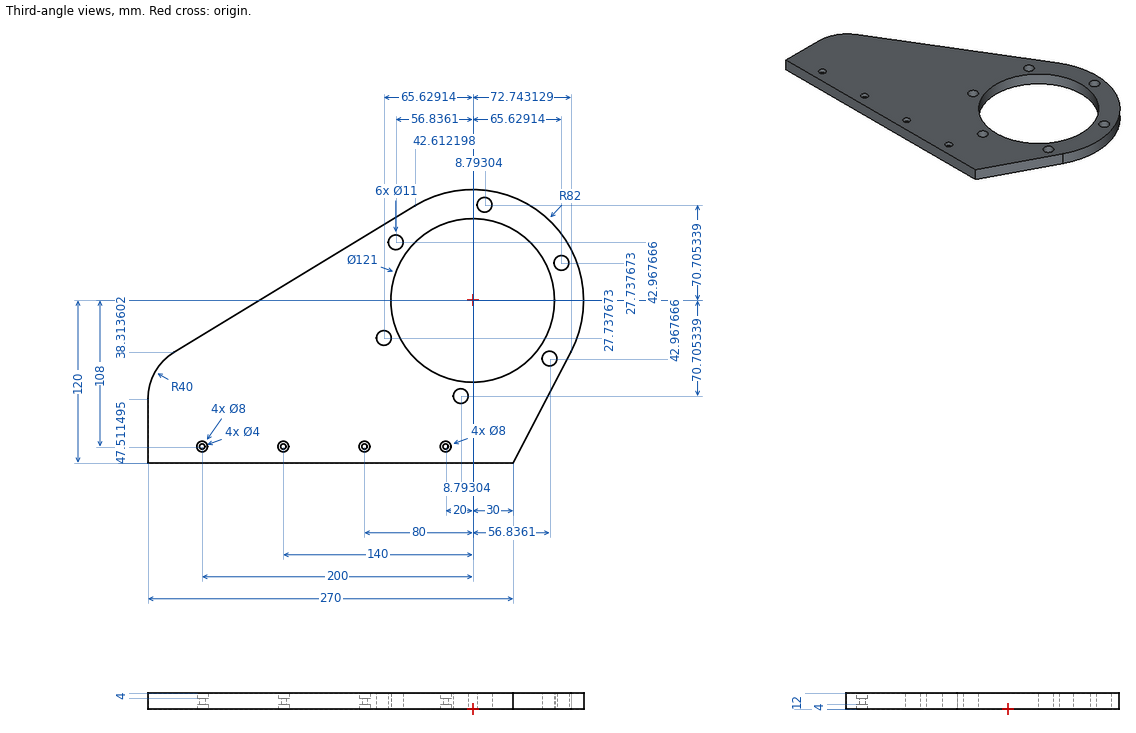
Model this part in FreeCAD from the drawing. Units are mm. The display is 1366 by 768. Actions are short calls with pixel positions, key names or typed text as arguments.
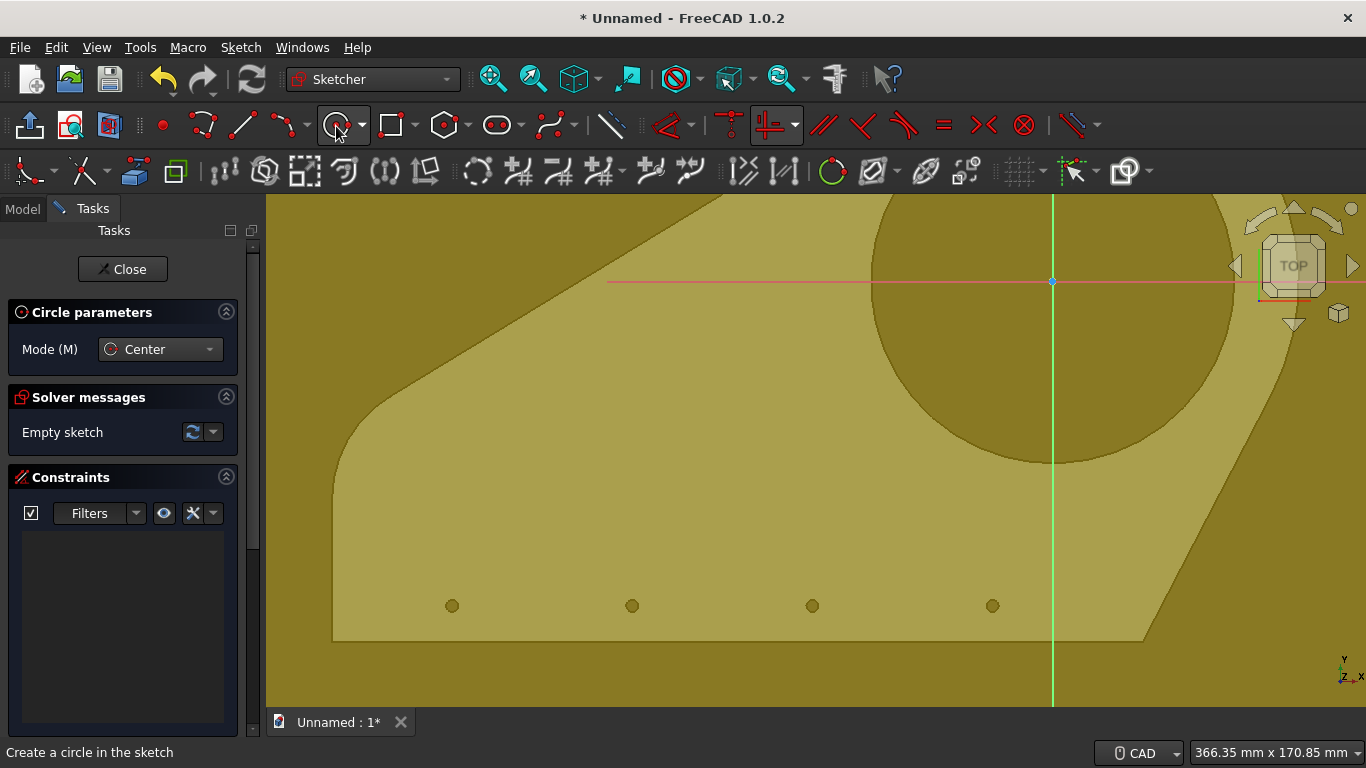
scroll(993, 606, up, 4)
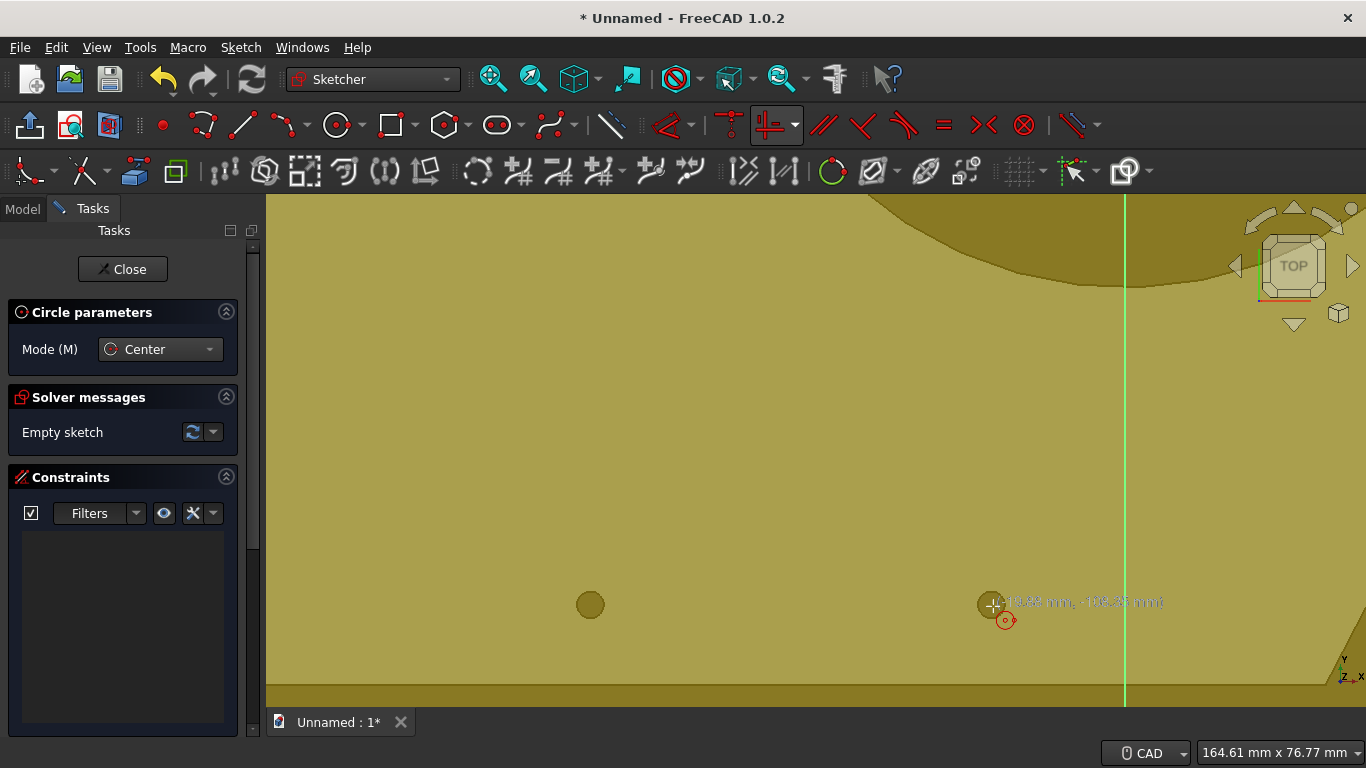
click(991, 605)
click(1010, 586)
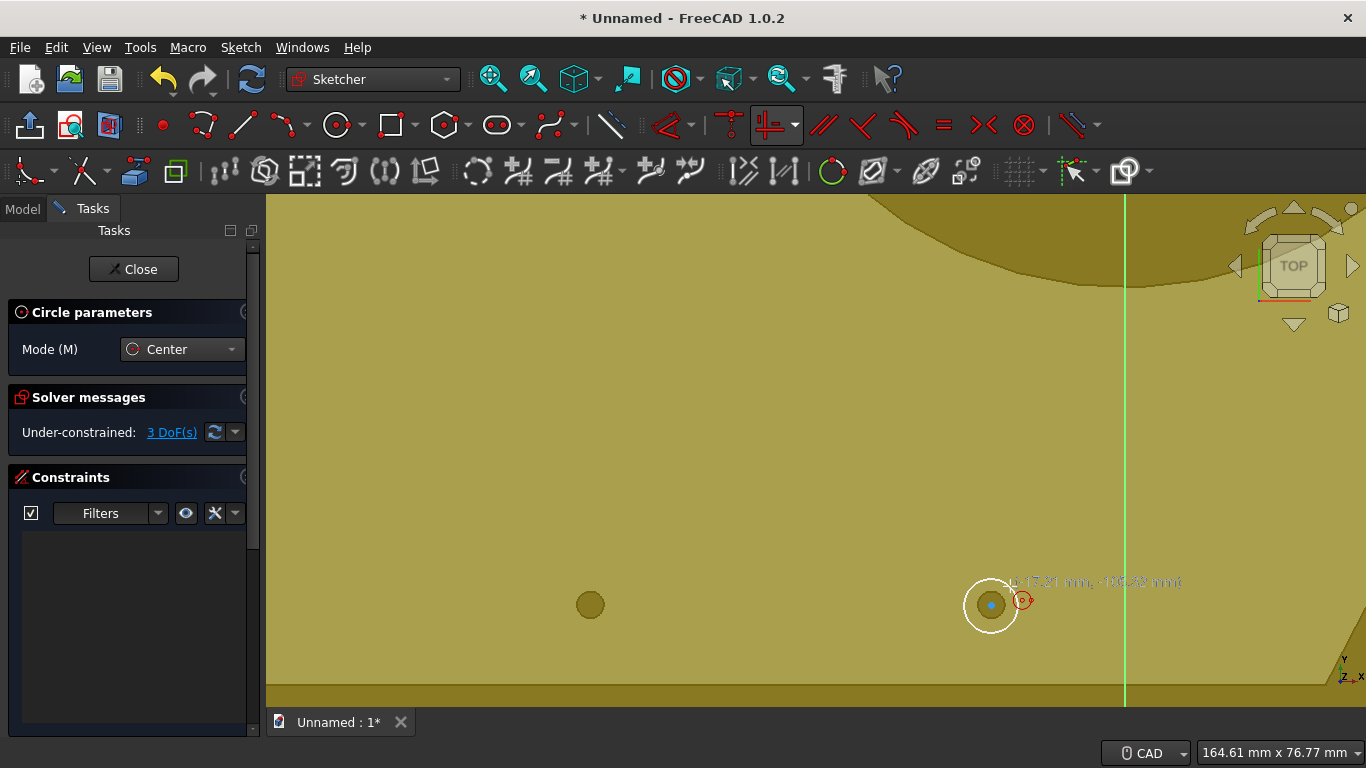
click(590, 605)
click(609, 586)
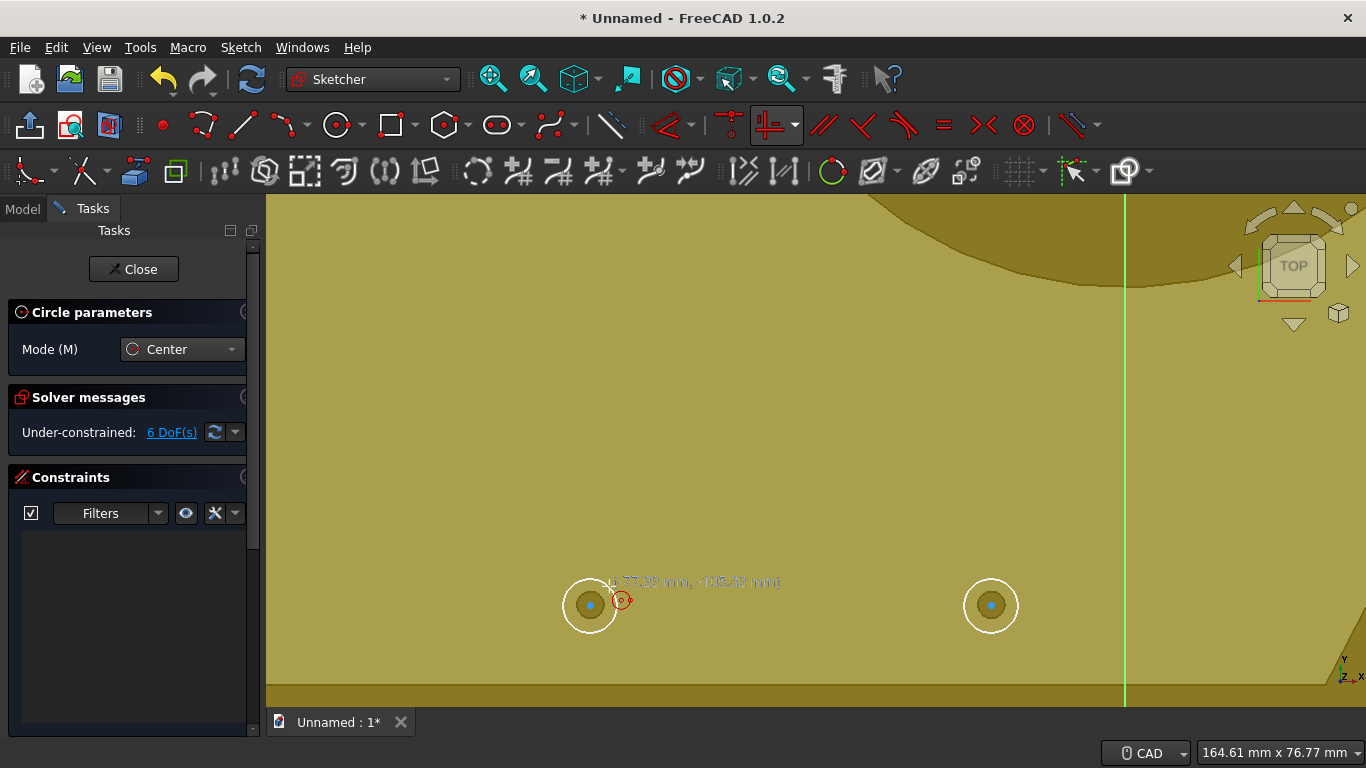
scroll(996, 608, down, 4)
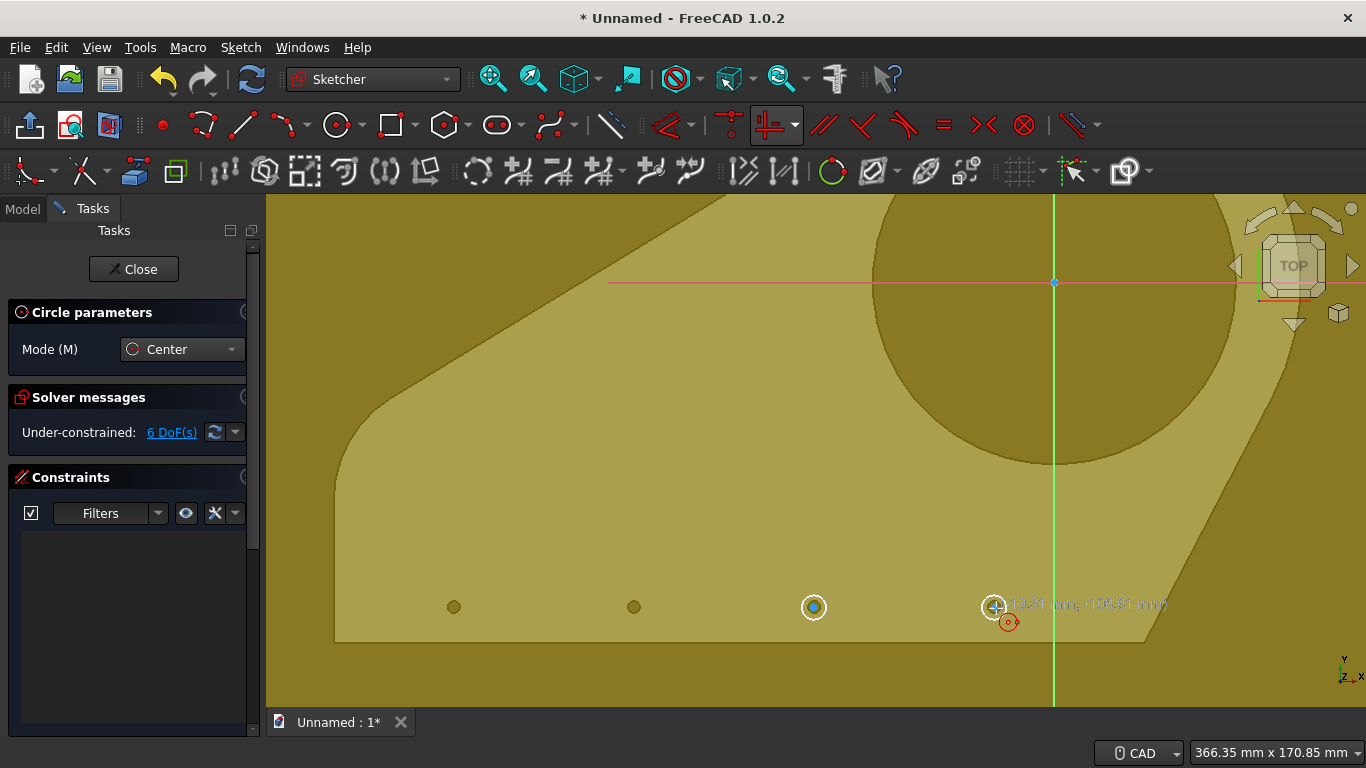
scroll(634, 607, up, 4)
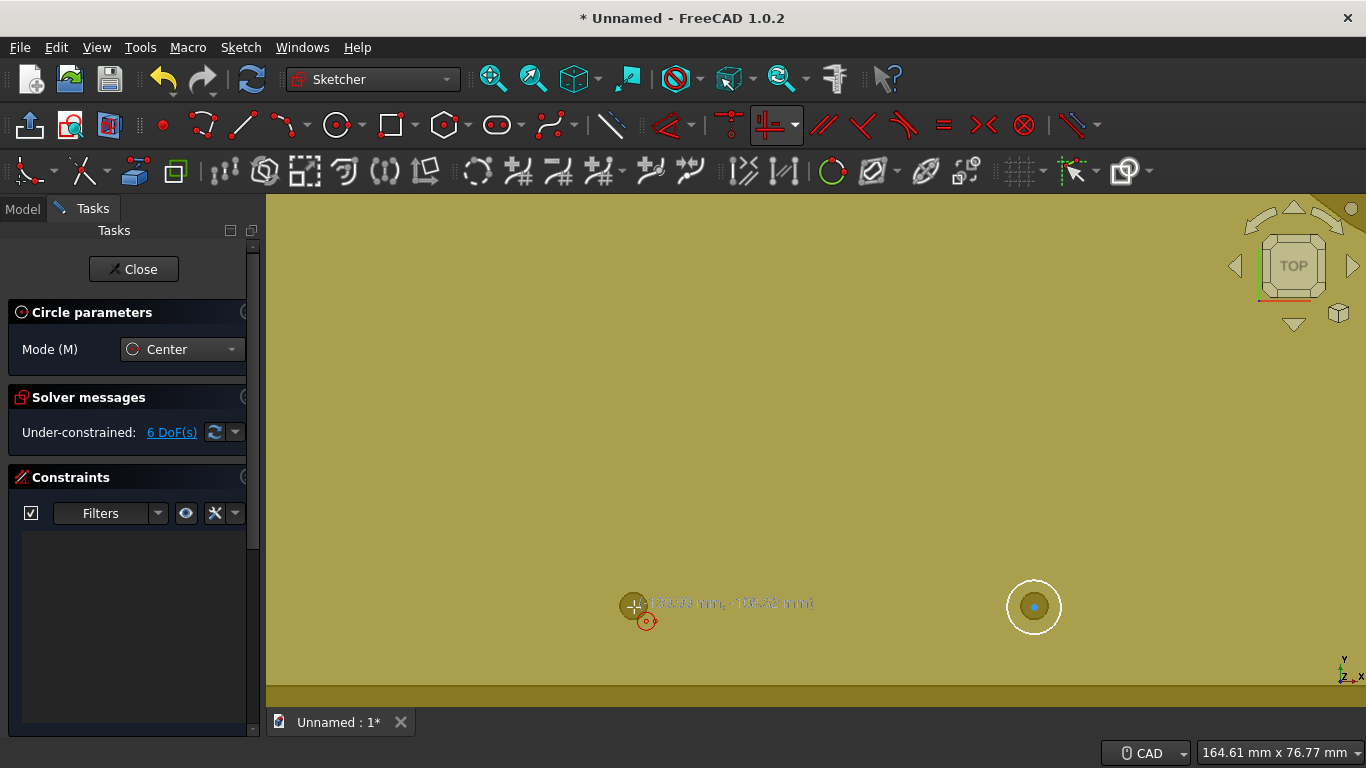
click(634, 606)
click(652, 587)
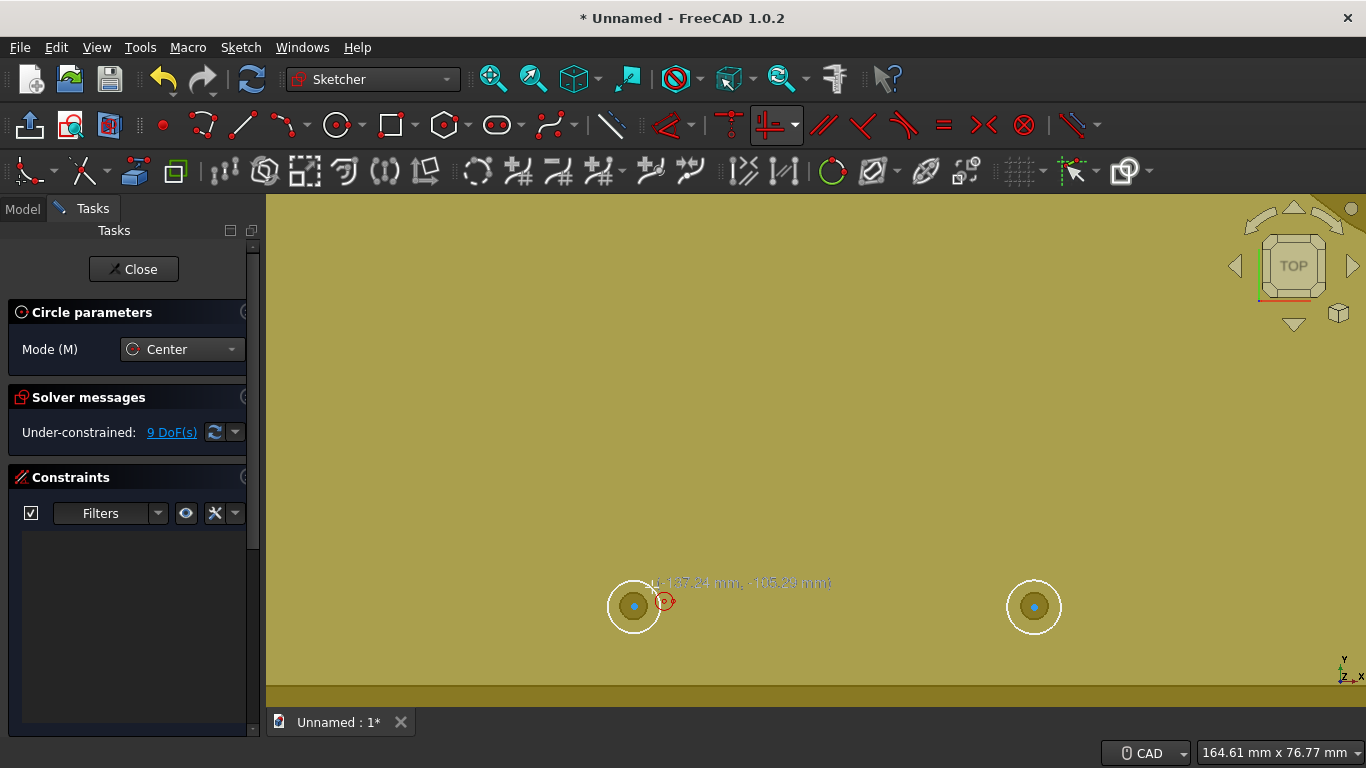
scroll(633, 607, down, 4)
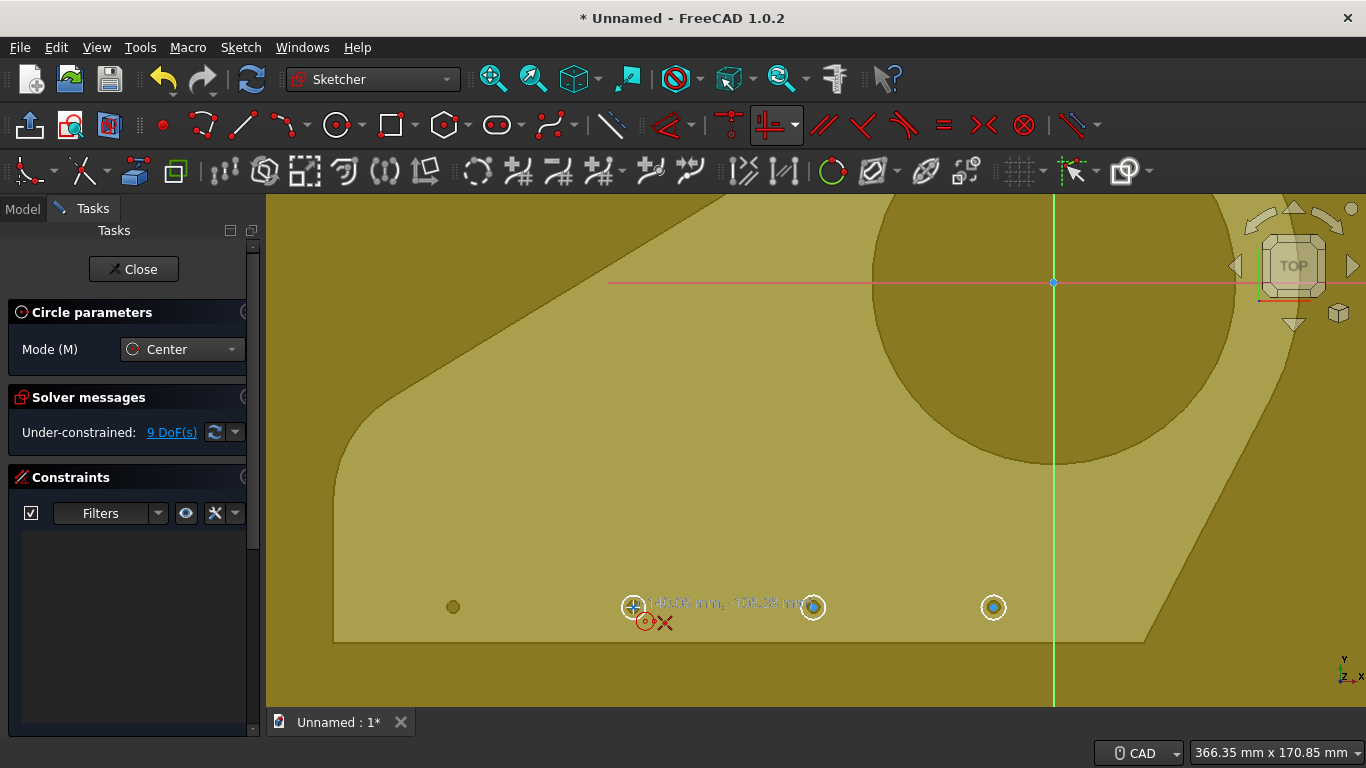
scroll(453, 607, up, 4)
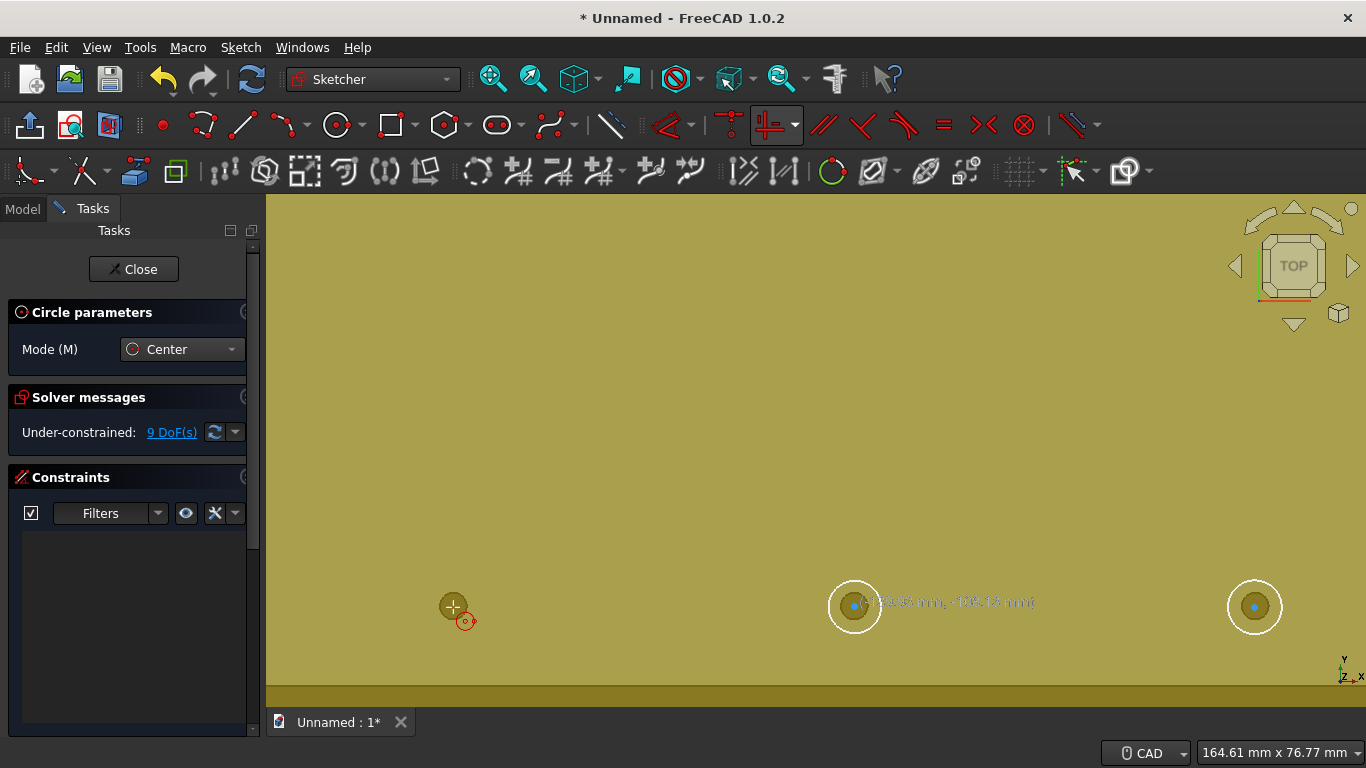
click(453, 606)
click(472, 587)
key(Escape)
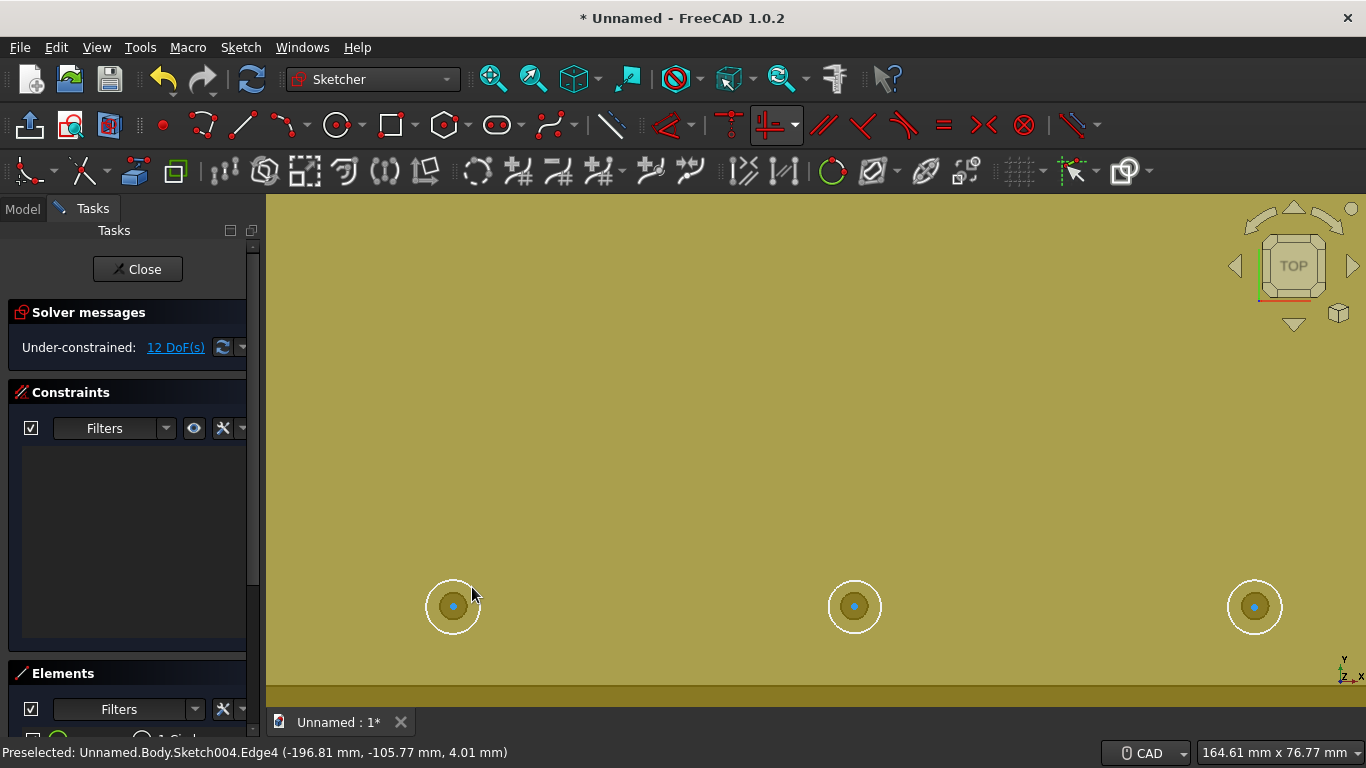
scroll(453, 607, down, 4)